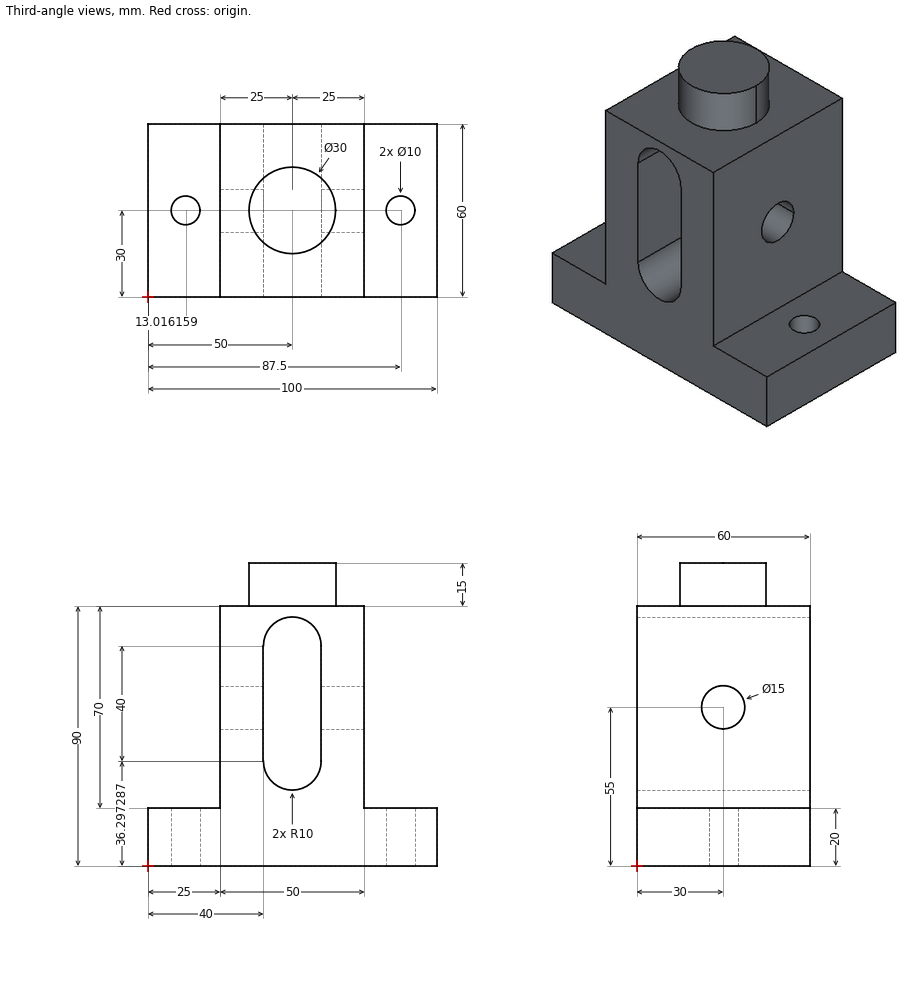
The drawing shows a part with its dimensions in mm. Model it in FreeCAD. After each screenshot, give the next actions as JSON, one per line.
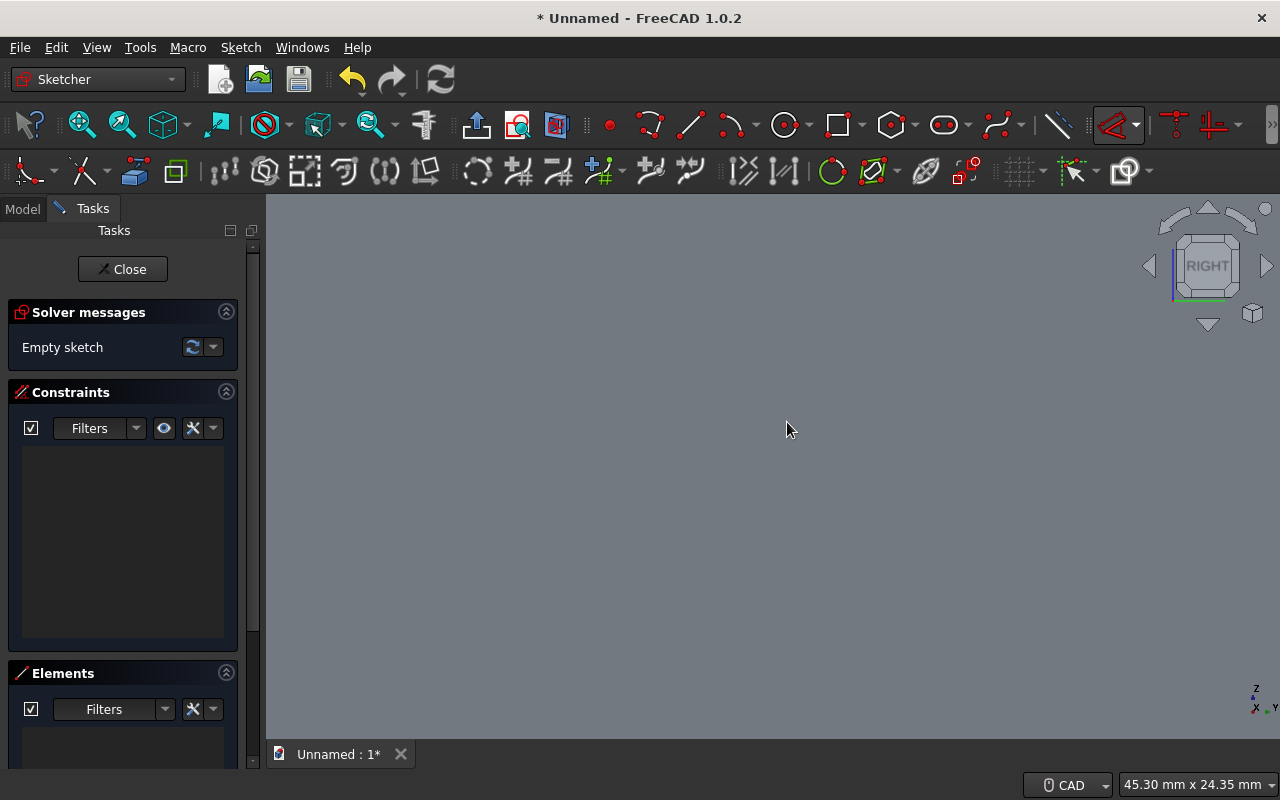
{"action": "key", "text": "g c"}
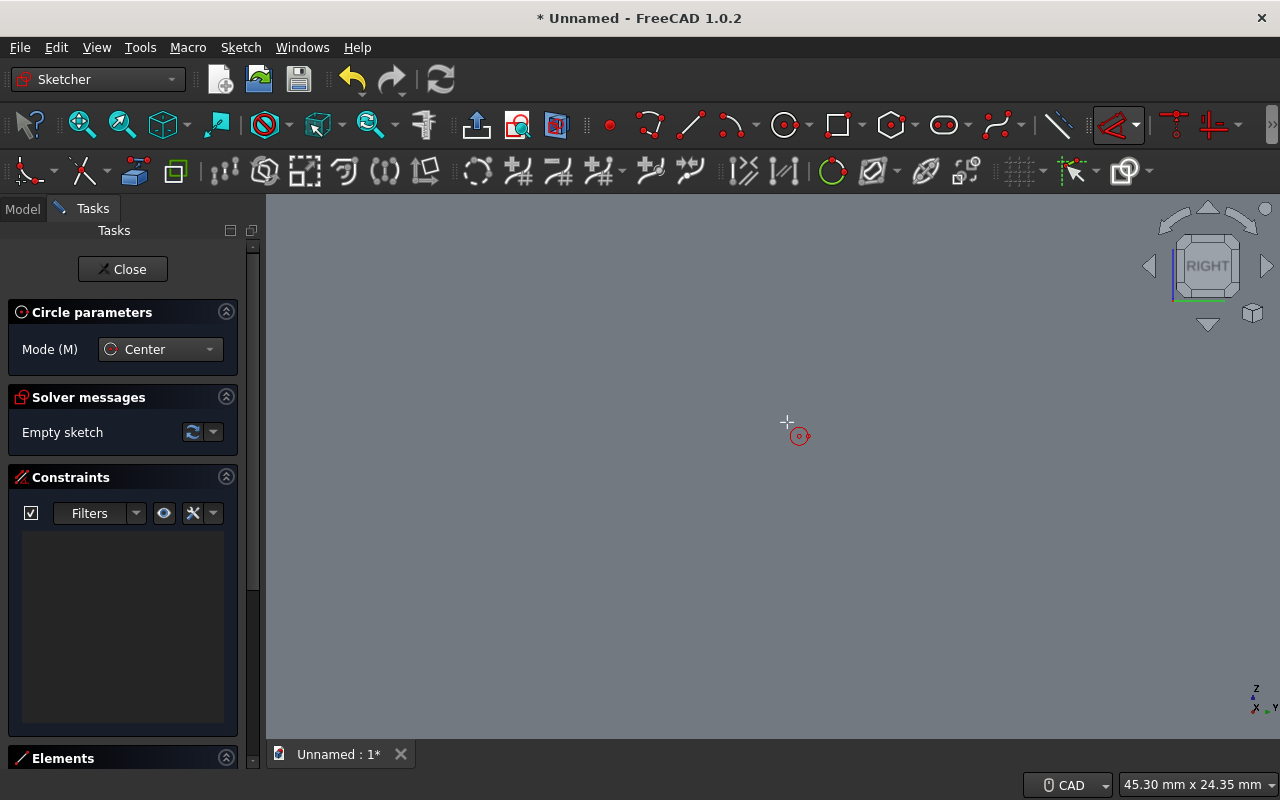
{"action": "left_click", "coordinate": [700, 465]}
{"action": "left_click", "coordinate": [818, 347]}
{"action": "key", "text": "Escape"}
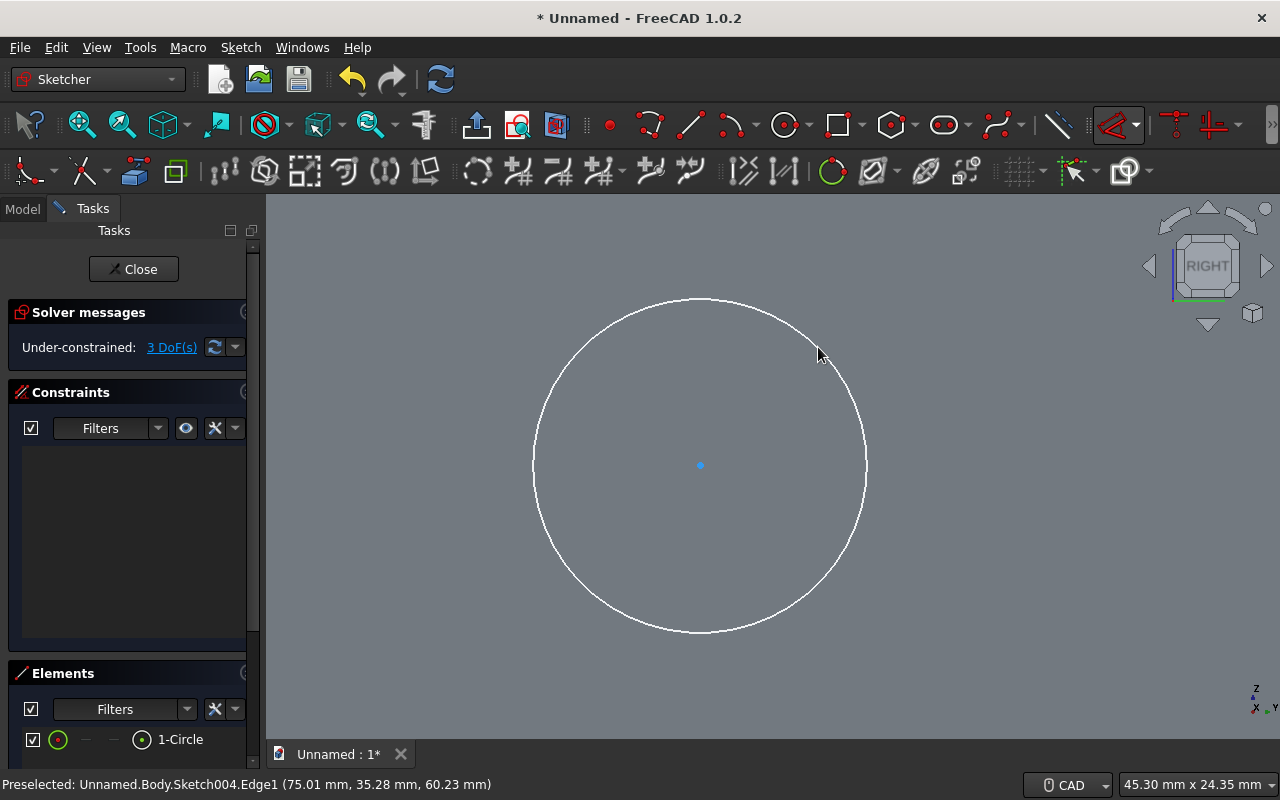
{"action": "left_click", "coordinate": [818, 348]}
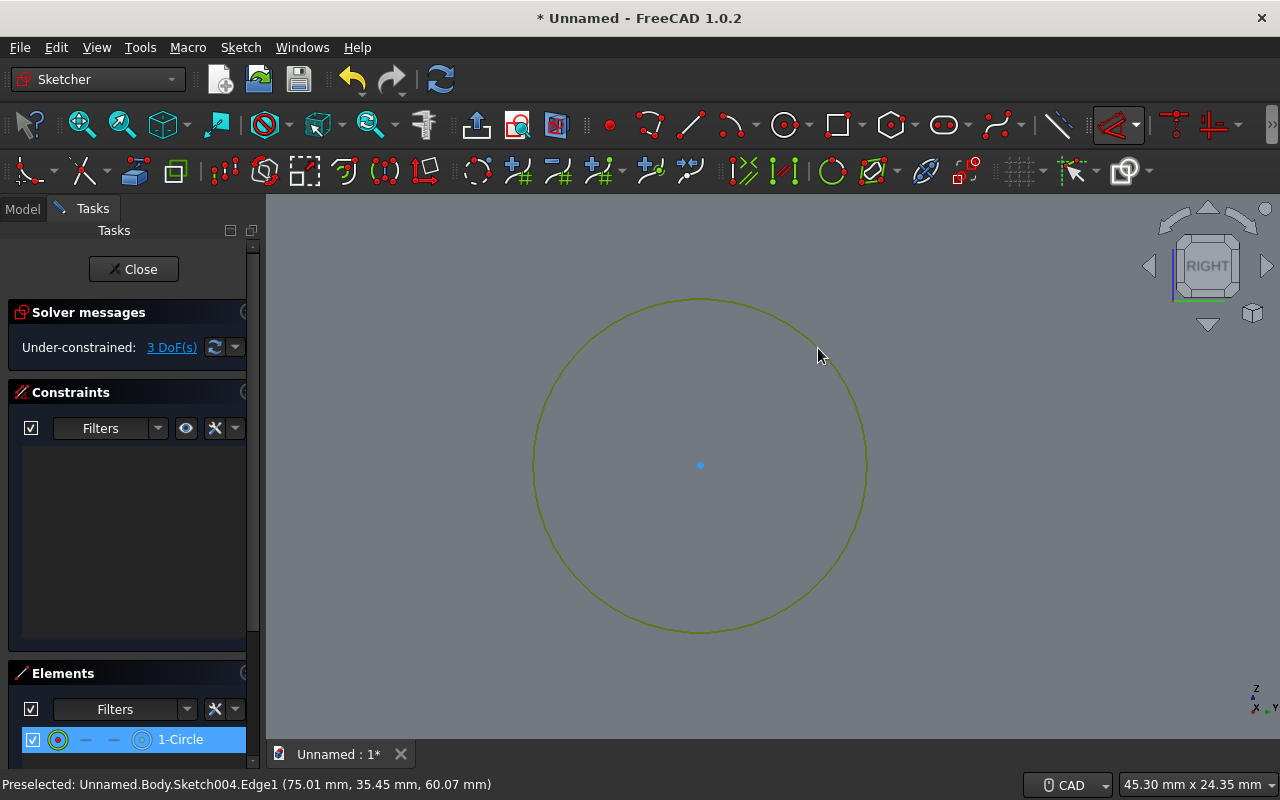
{"action": "key", "text": "k o"}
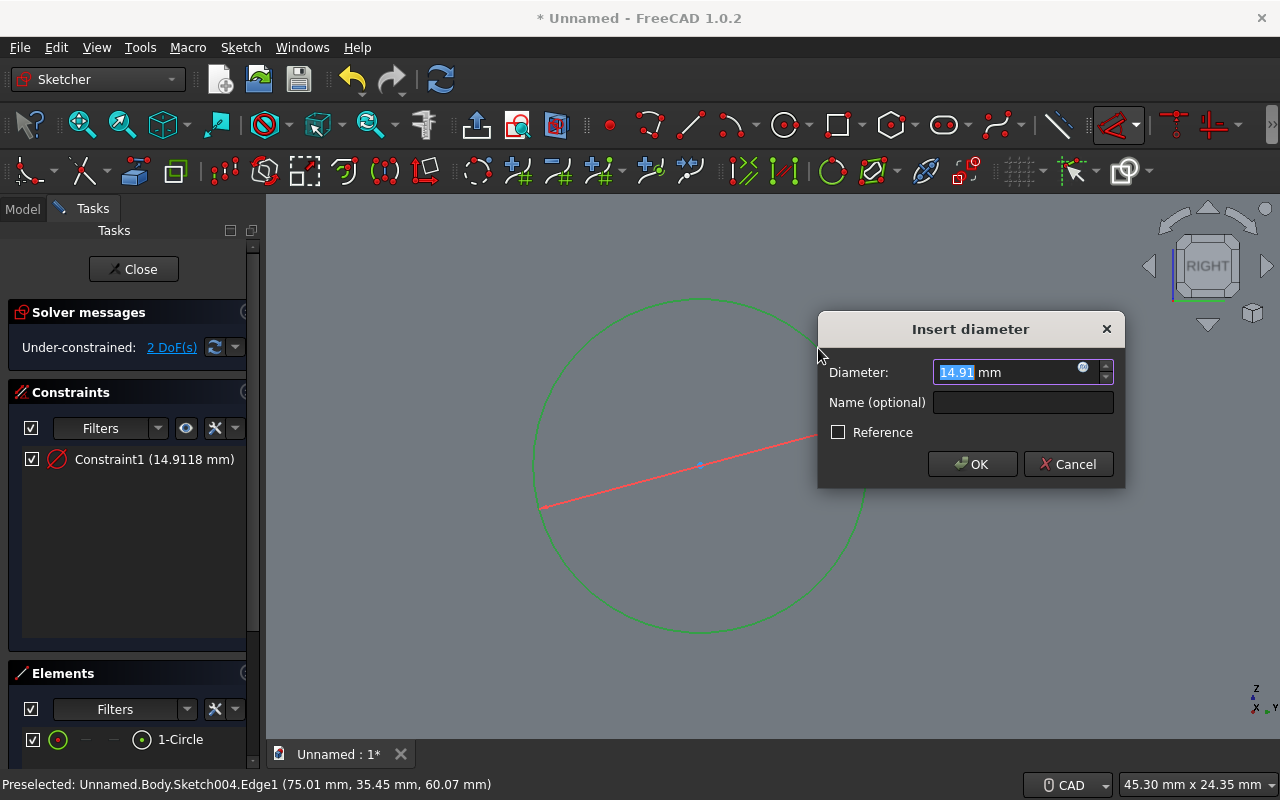
{"action": "type", "text": "15"}
{"action": "key", "text": "Return"}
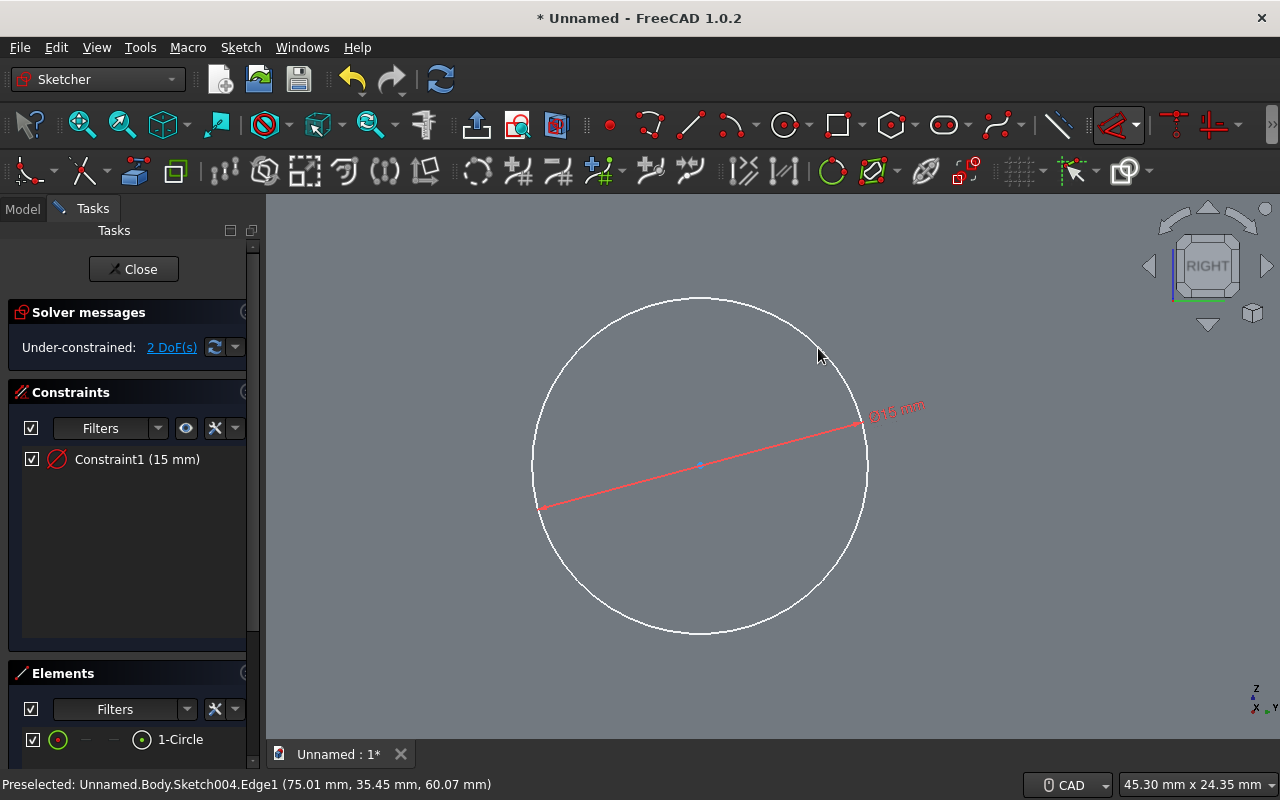
{"action": "left_click", "coordinate": [700, 466]}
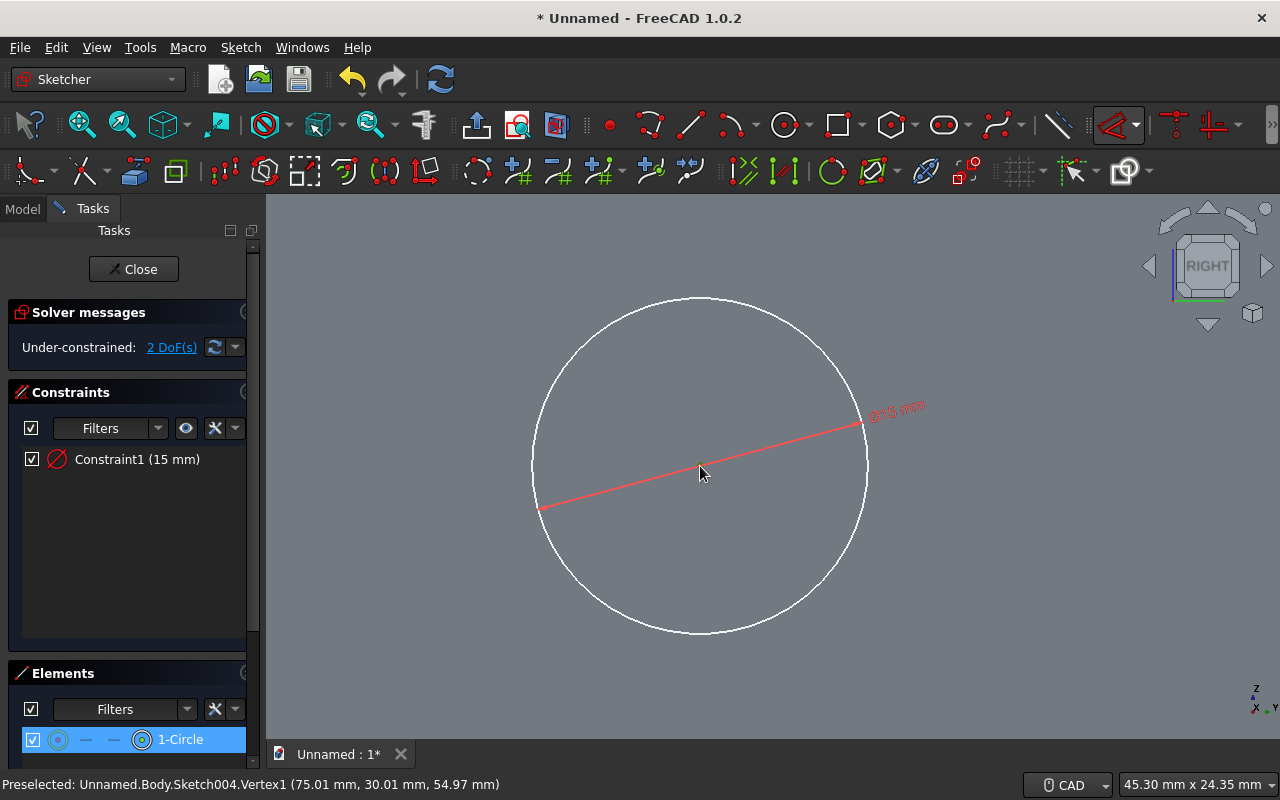
{"action": "key", "text": "l"}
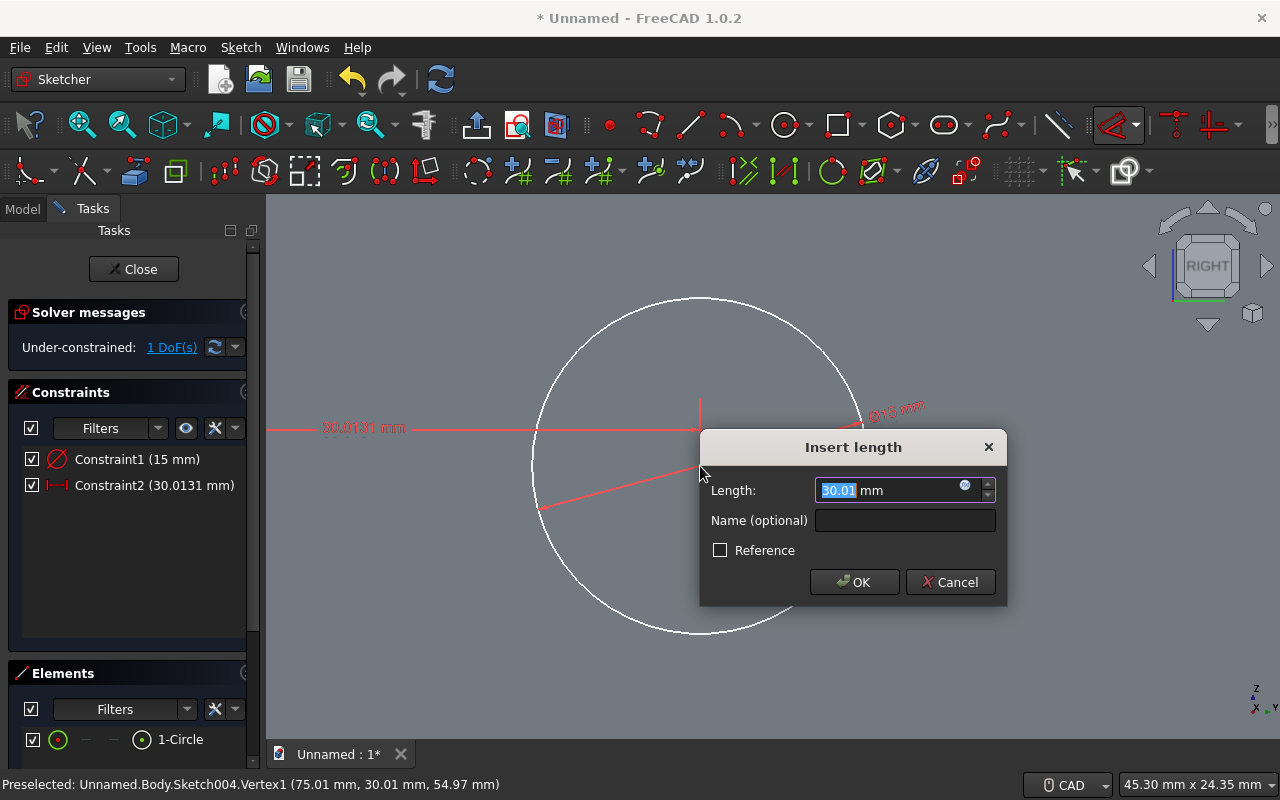
{"action": "type", "text": "30"}
{"action": "key", "text": "Return"}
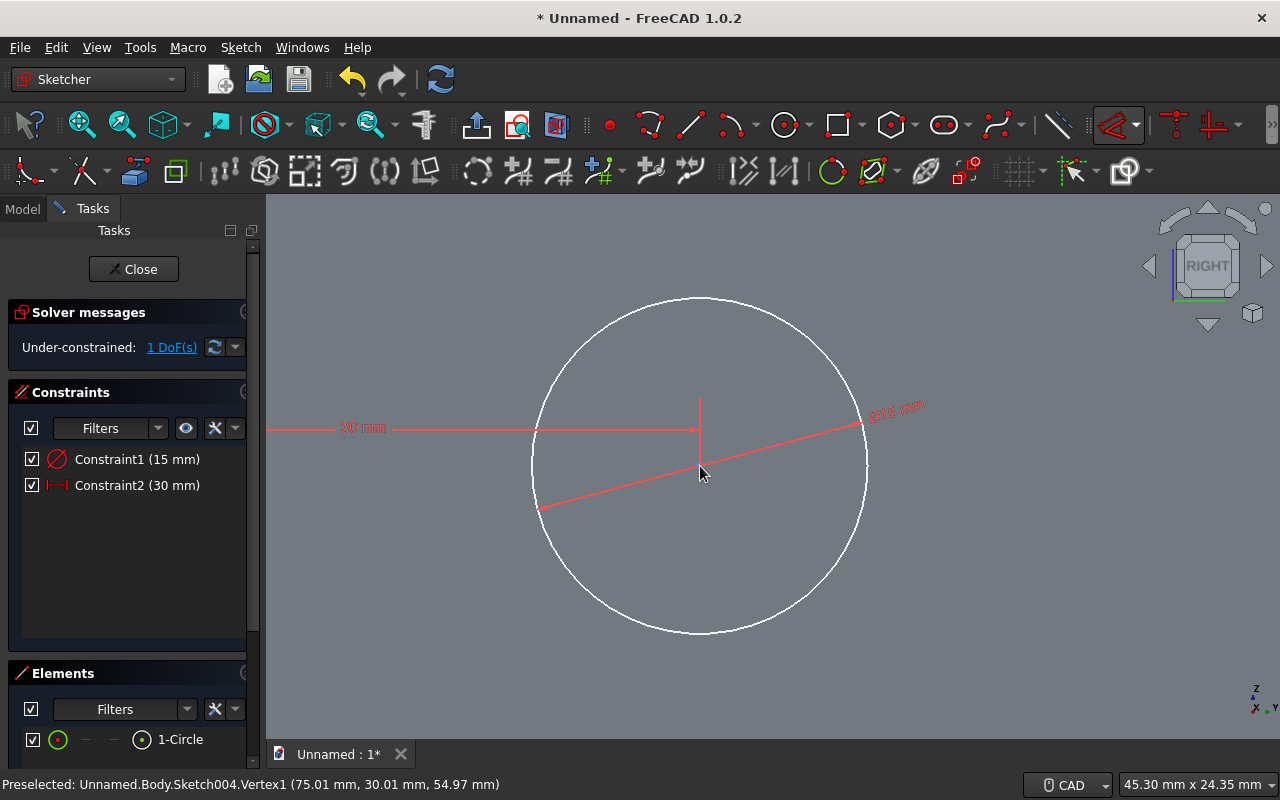
{"action": "left_click", "coordinate": [700, 466]}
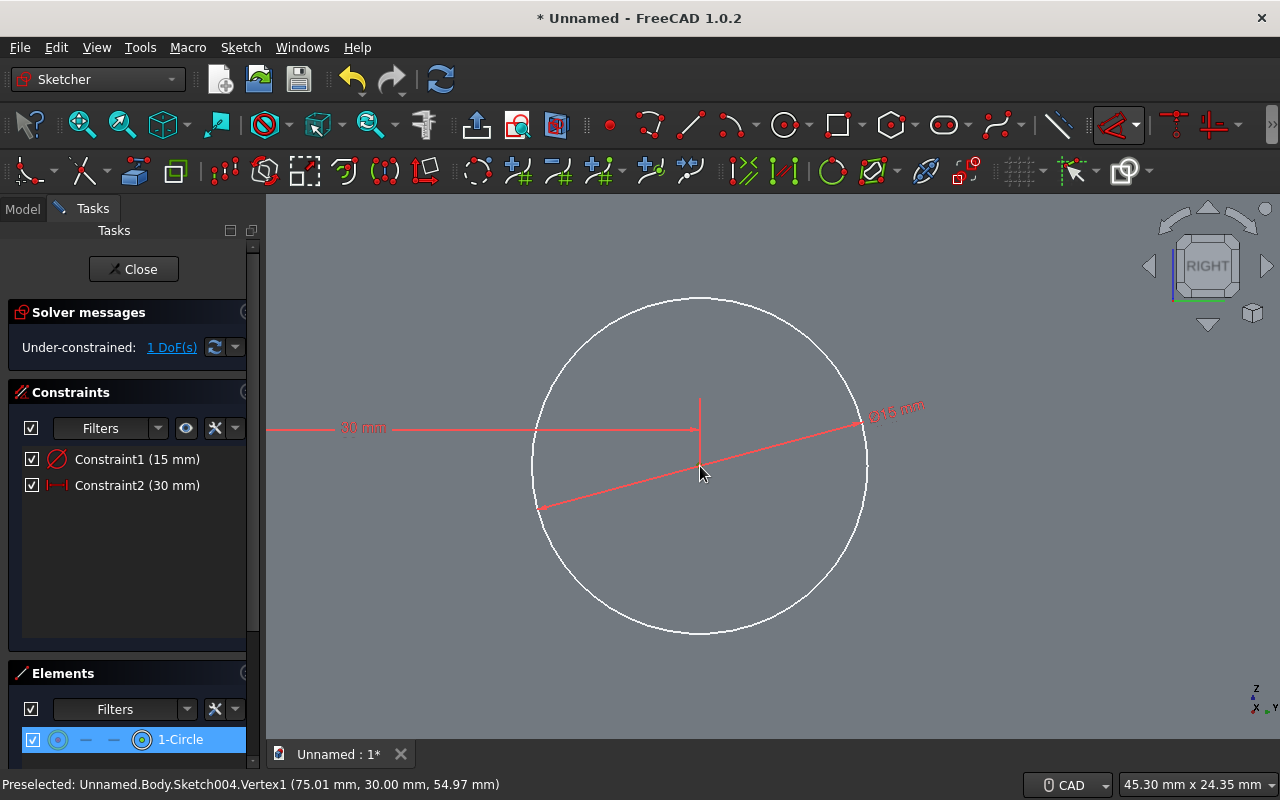
{"action": "key", "text": "i"}